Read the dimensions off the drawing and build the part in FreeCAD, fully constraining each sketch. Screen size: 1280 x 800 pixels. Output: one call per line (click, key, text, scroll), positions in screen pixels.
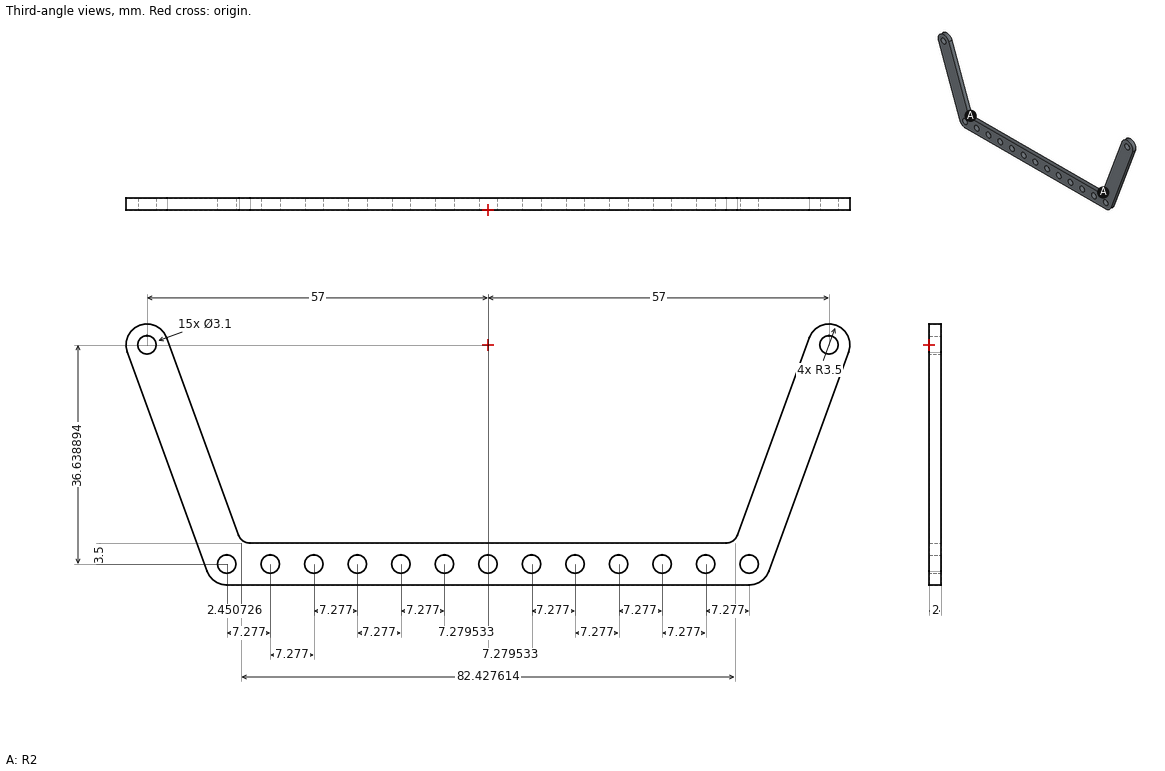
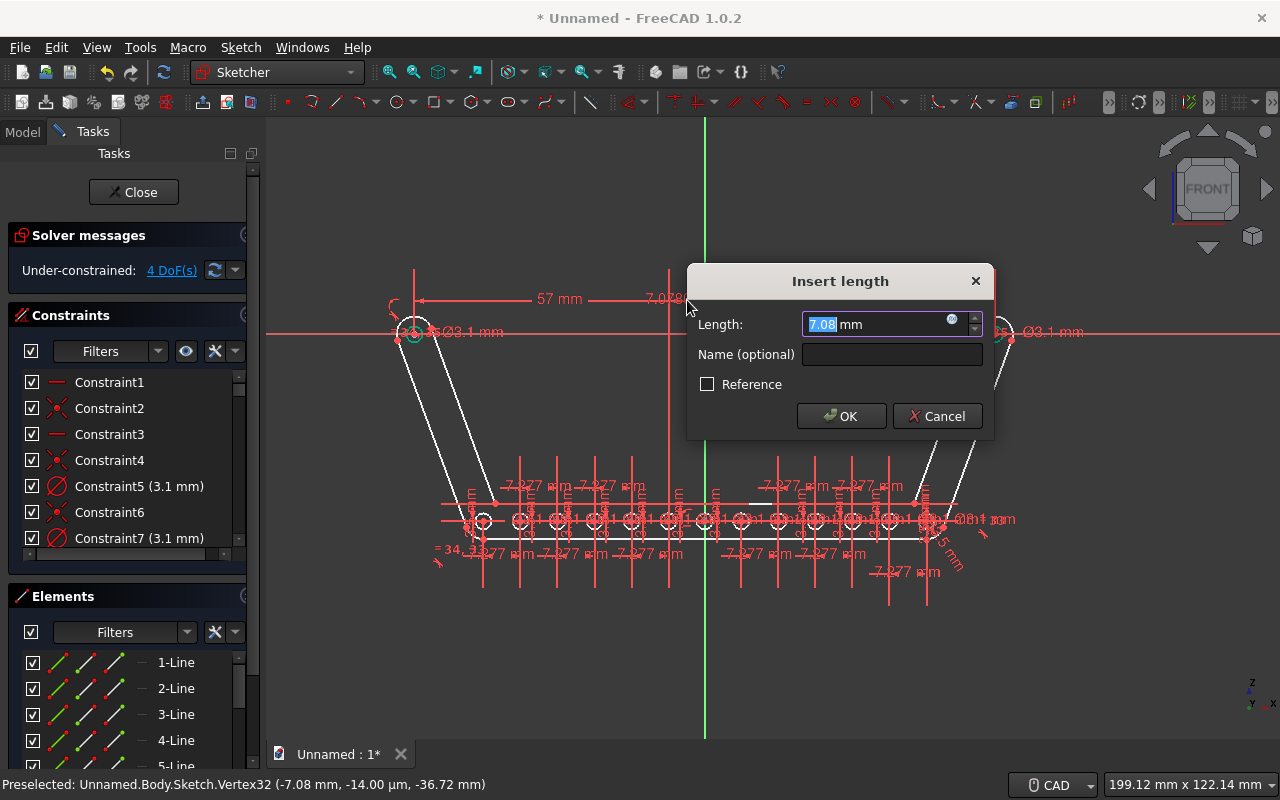
text(7.279533)
key(Return)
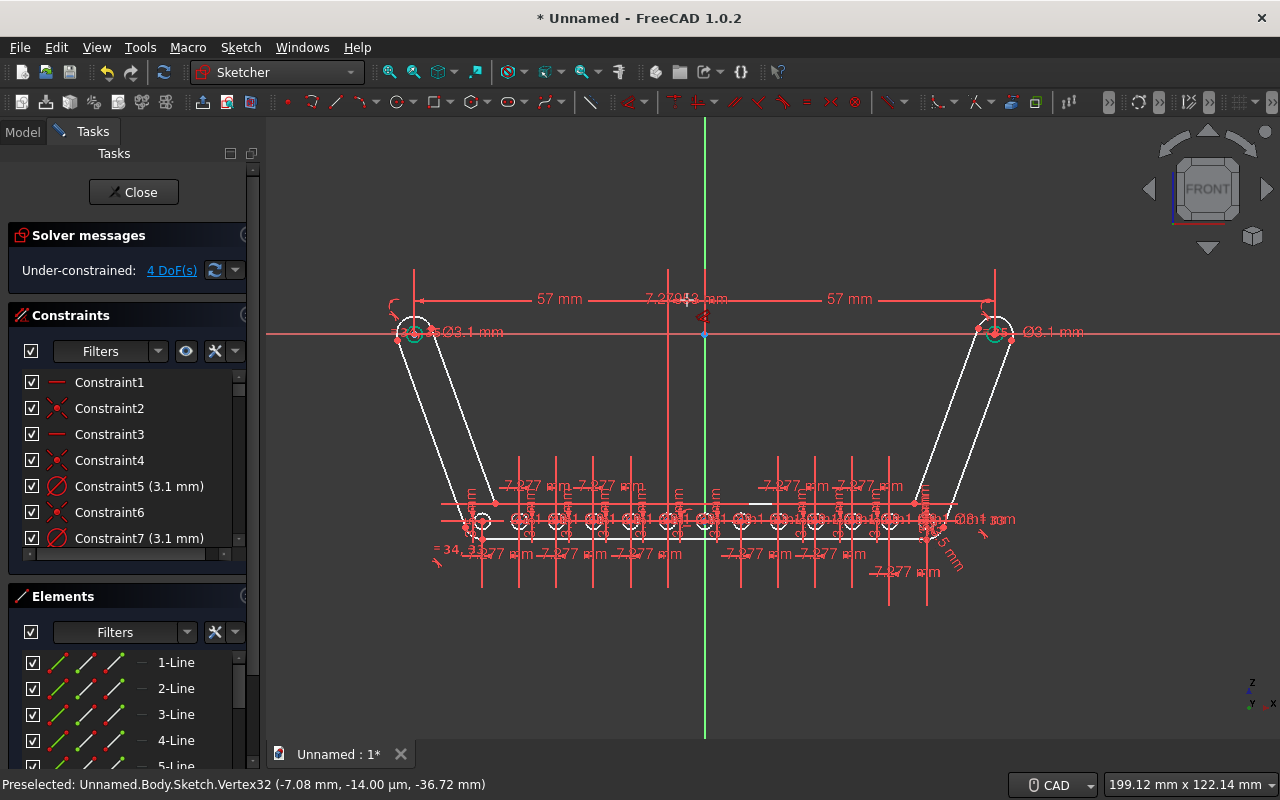
click(741, 521)
click(723, 276)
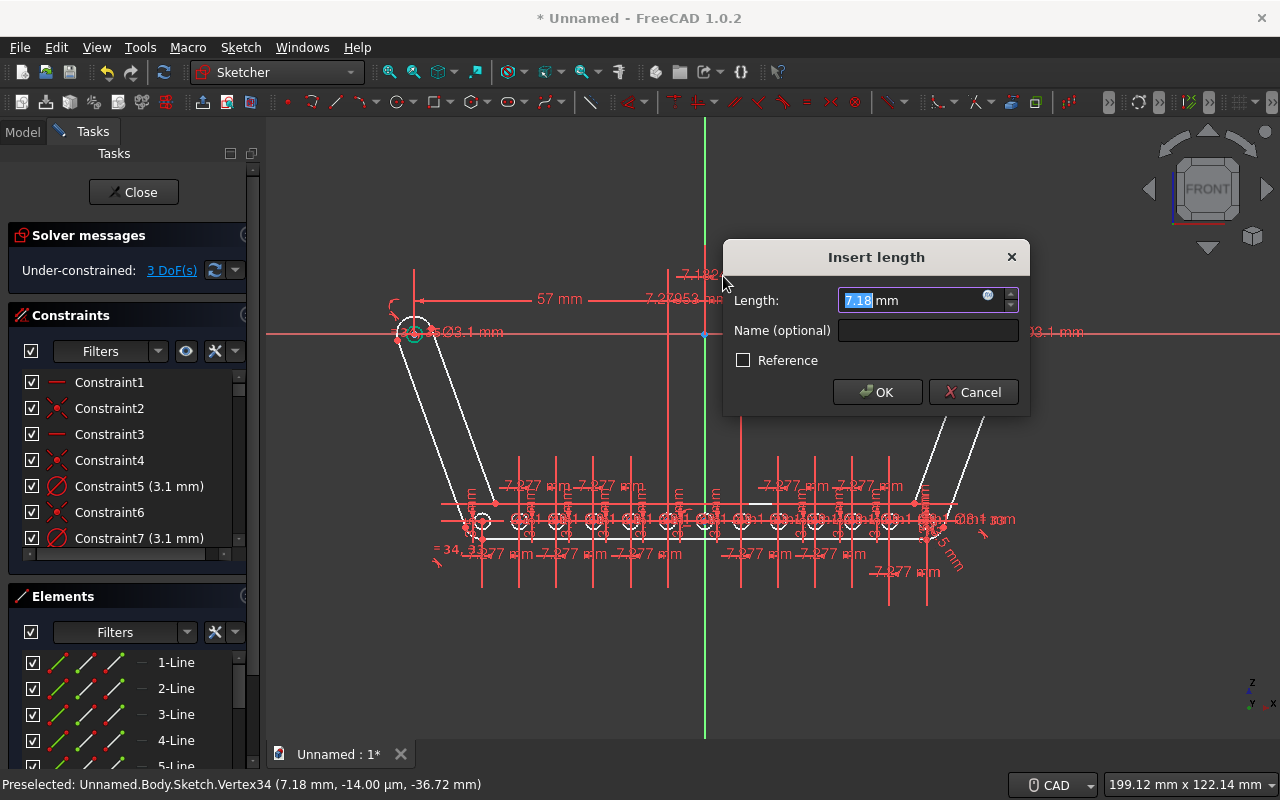
text(7.279533)
key(Return)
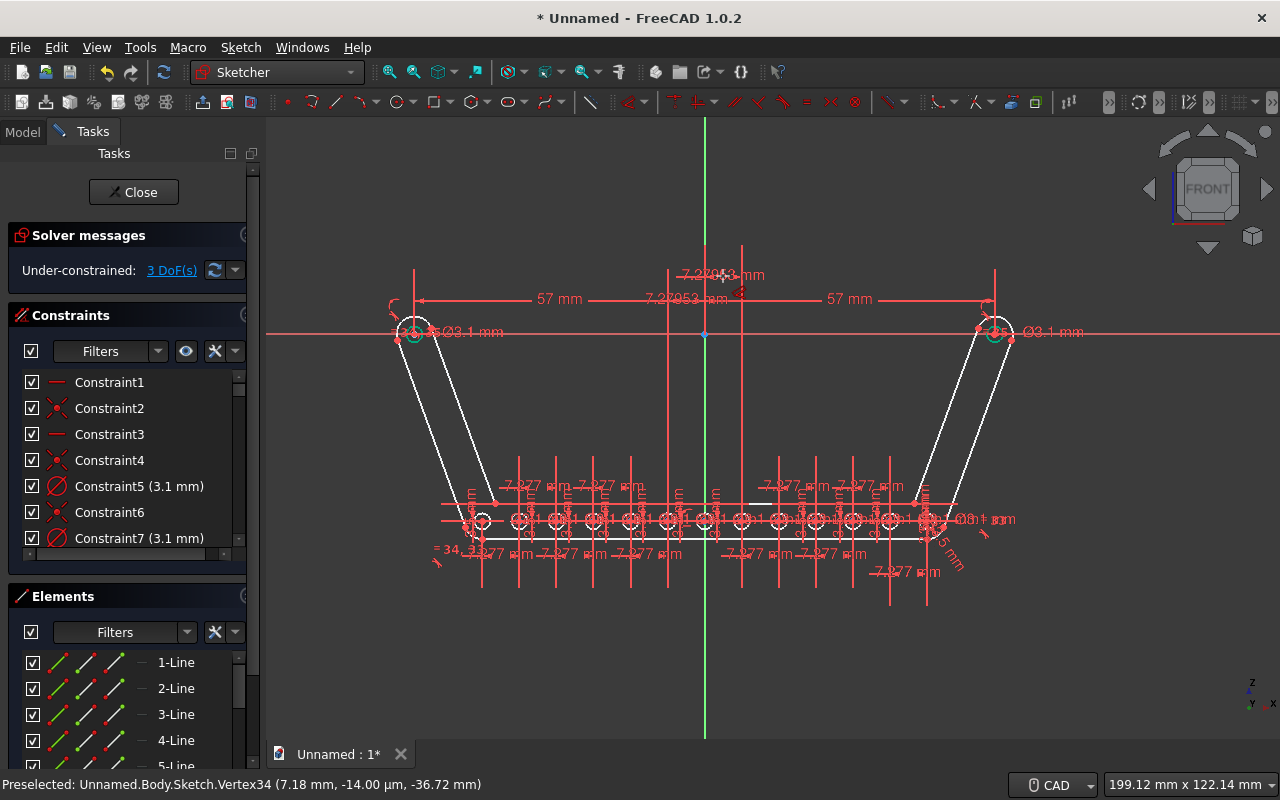
click(621, 504)
click(608, 446)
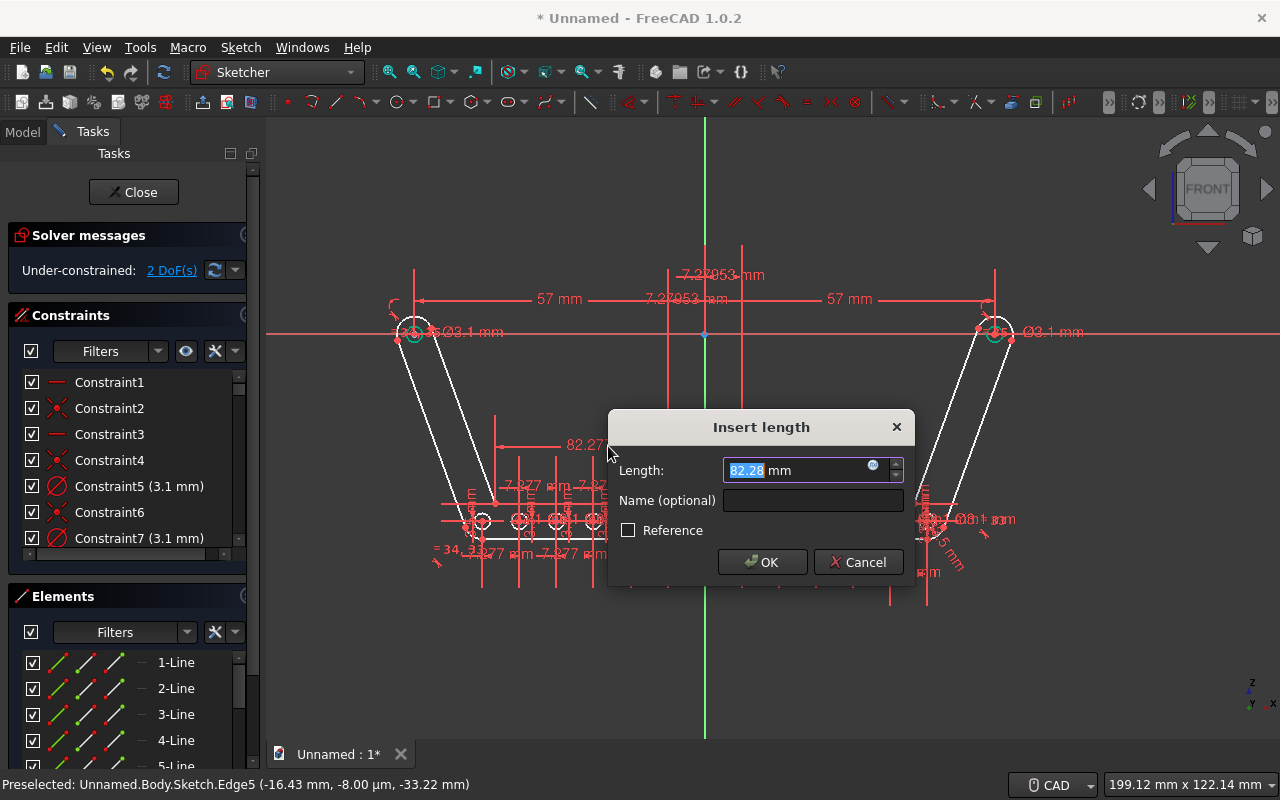
text(82.427614)
key(Return)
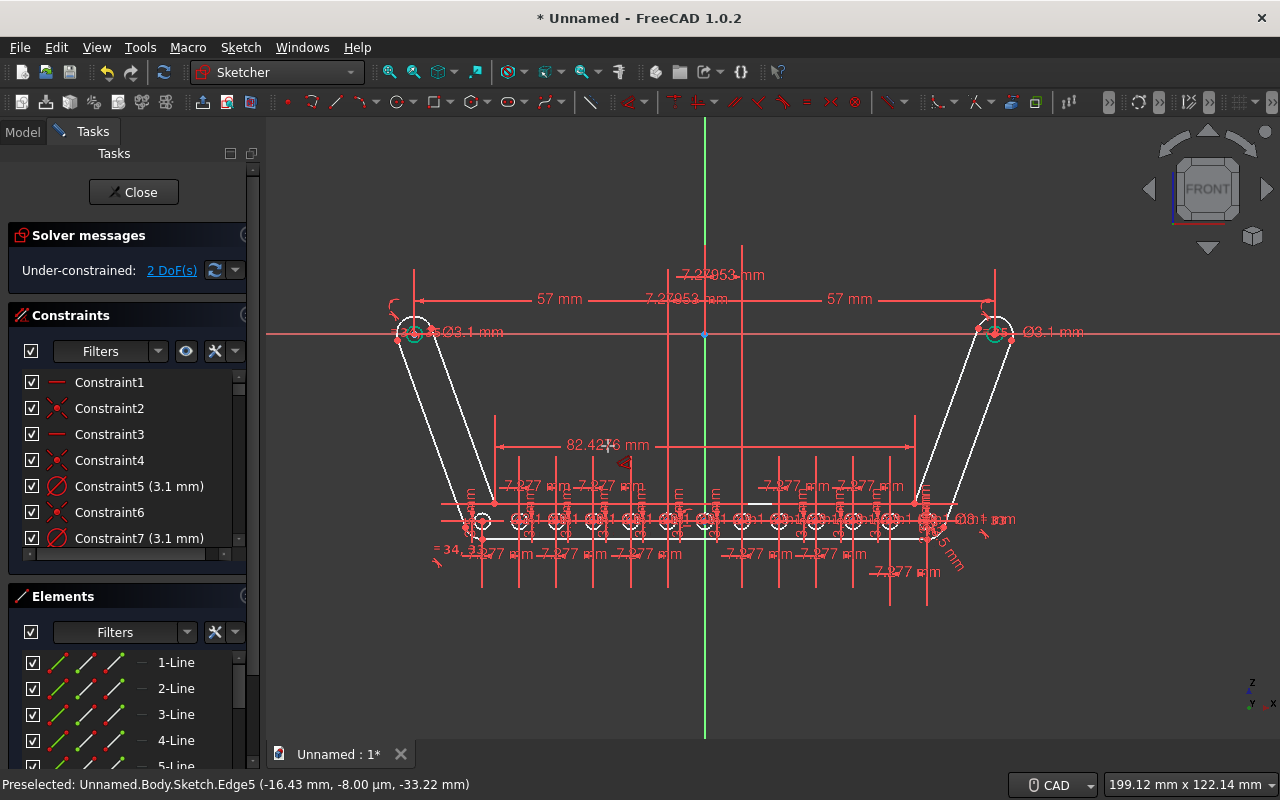
click(482, 521)
click(448, 428)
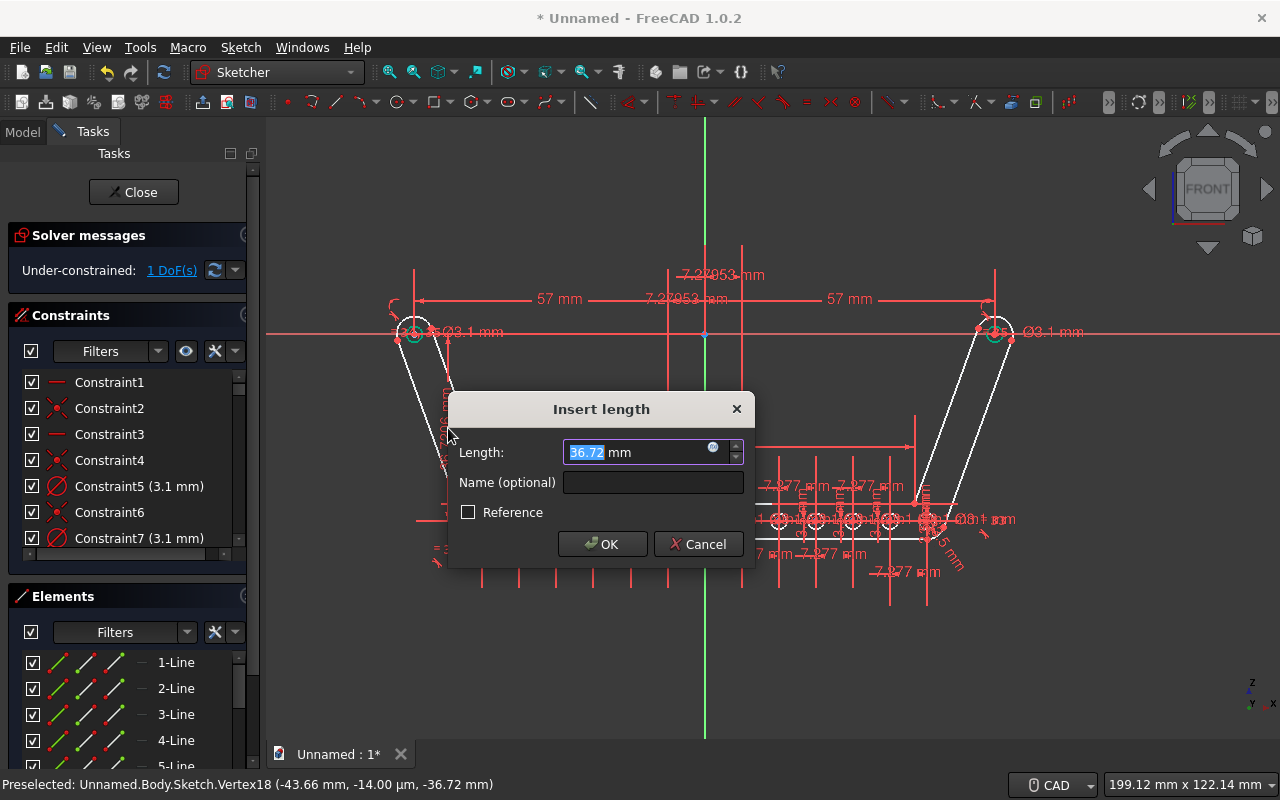
text(36.638894)
key(Return)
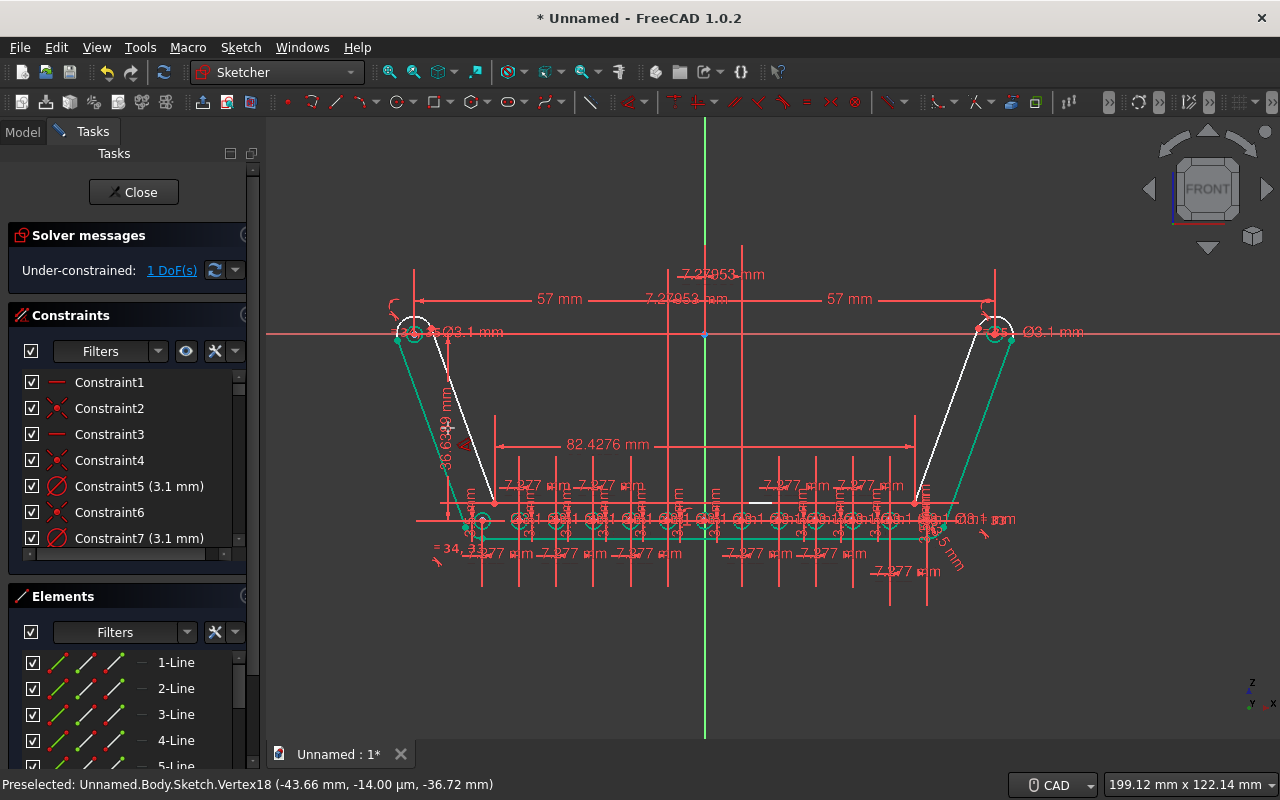
scroll(495, 503, up, 6)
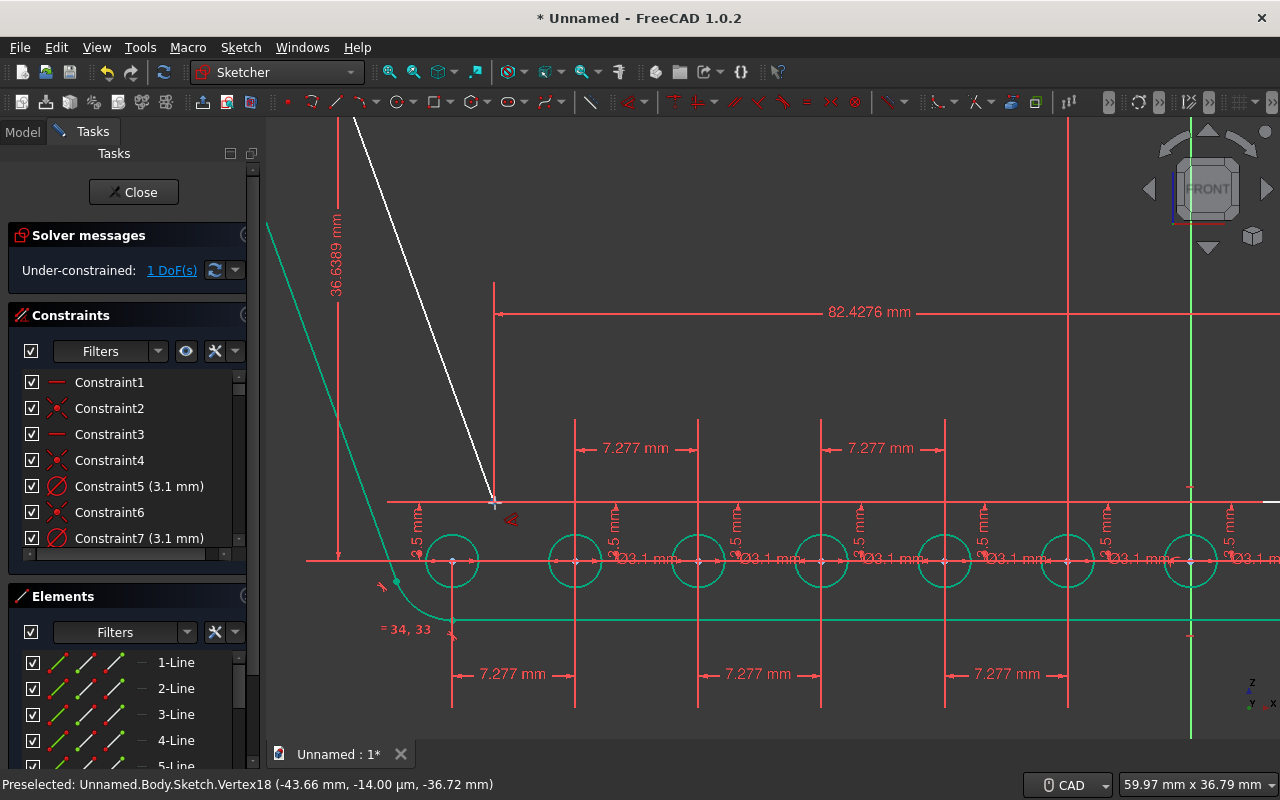
click(494, 502)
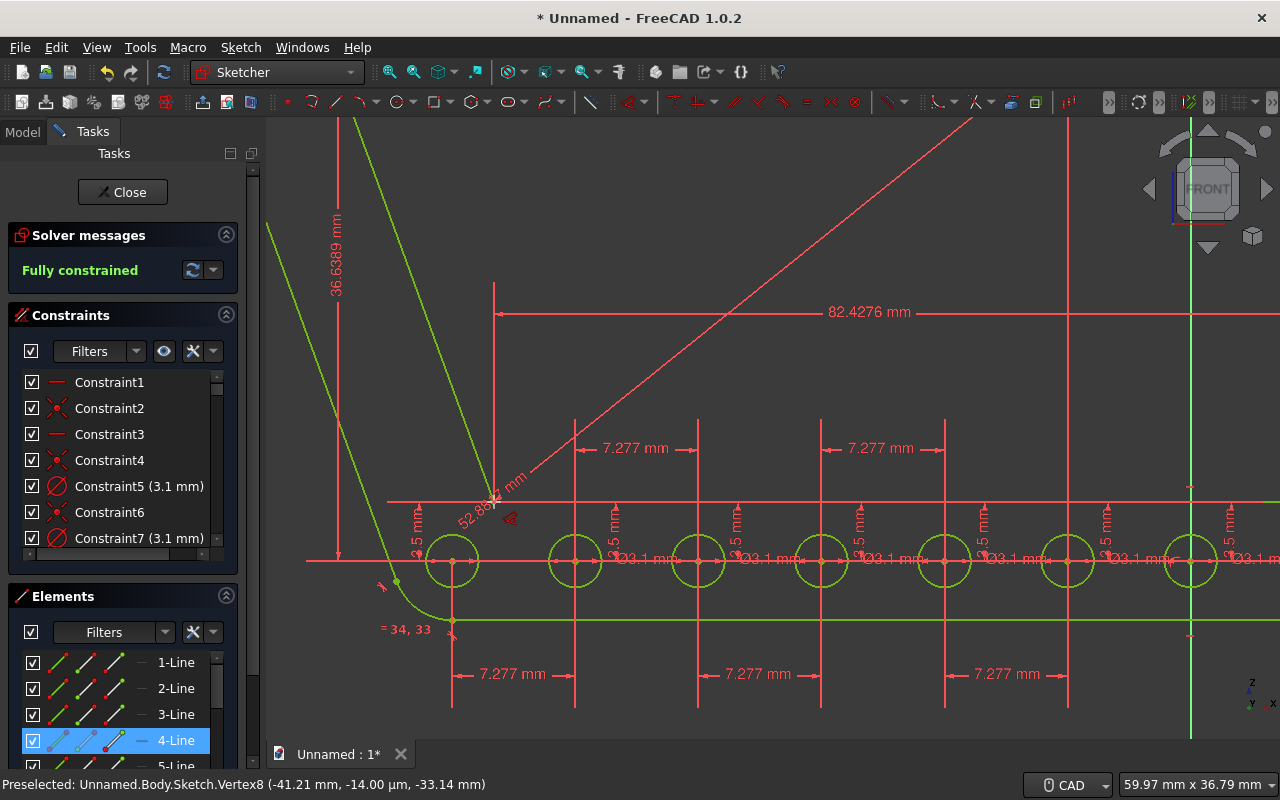
click(452, 561)
click(473, 595)